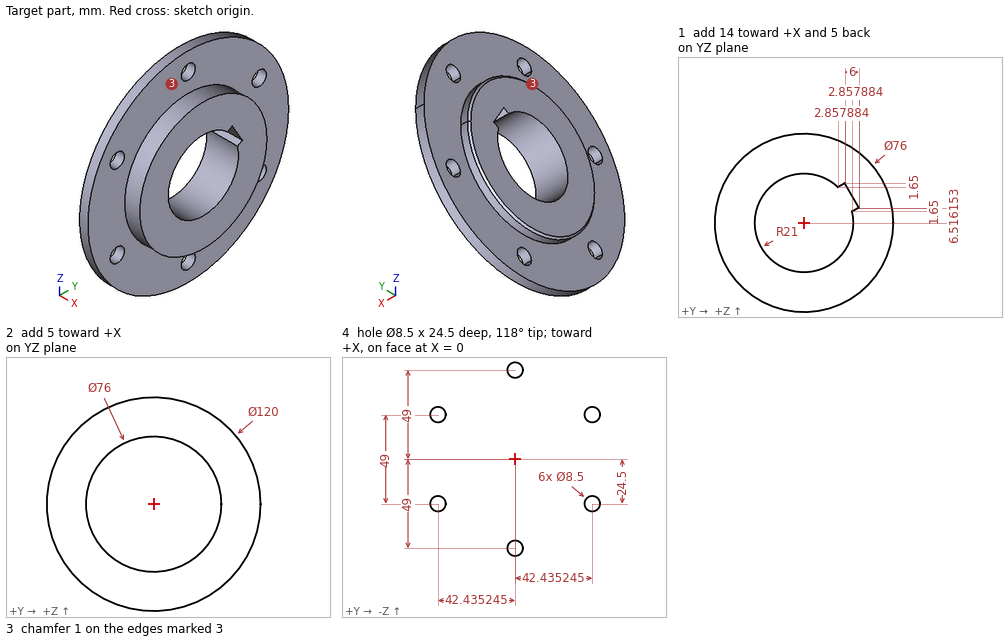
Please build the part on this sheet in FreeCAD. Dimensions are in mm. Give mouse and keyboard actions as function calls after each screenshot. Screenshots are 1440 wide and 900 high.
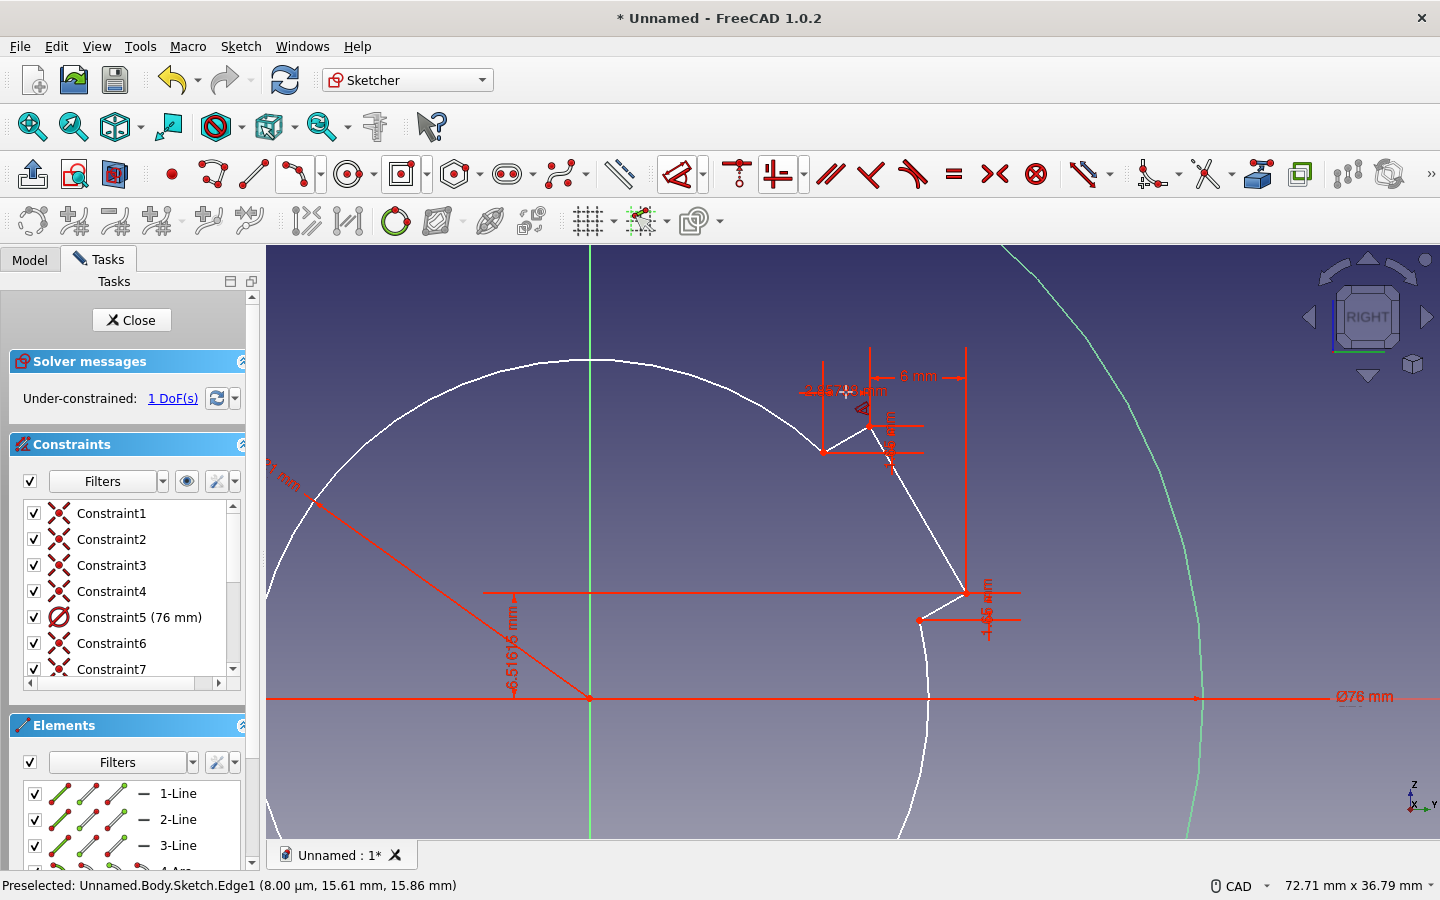
click(952, 601)
click(927, 559)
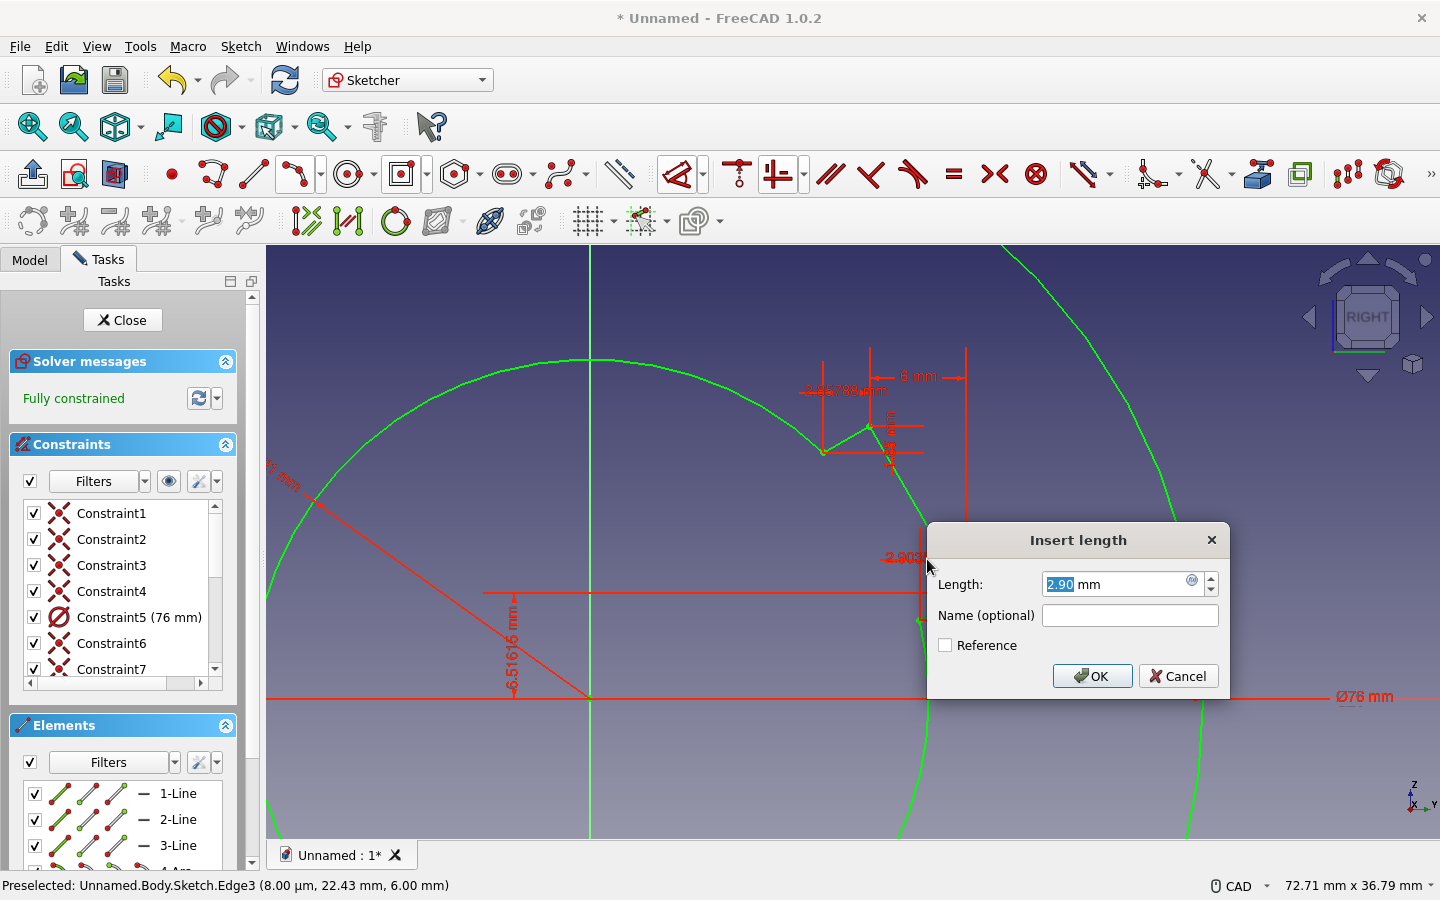
text(2.857884)
key(Return)
key(Escape)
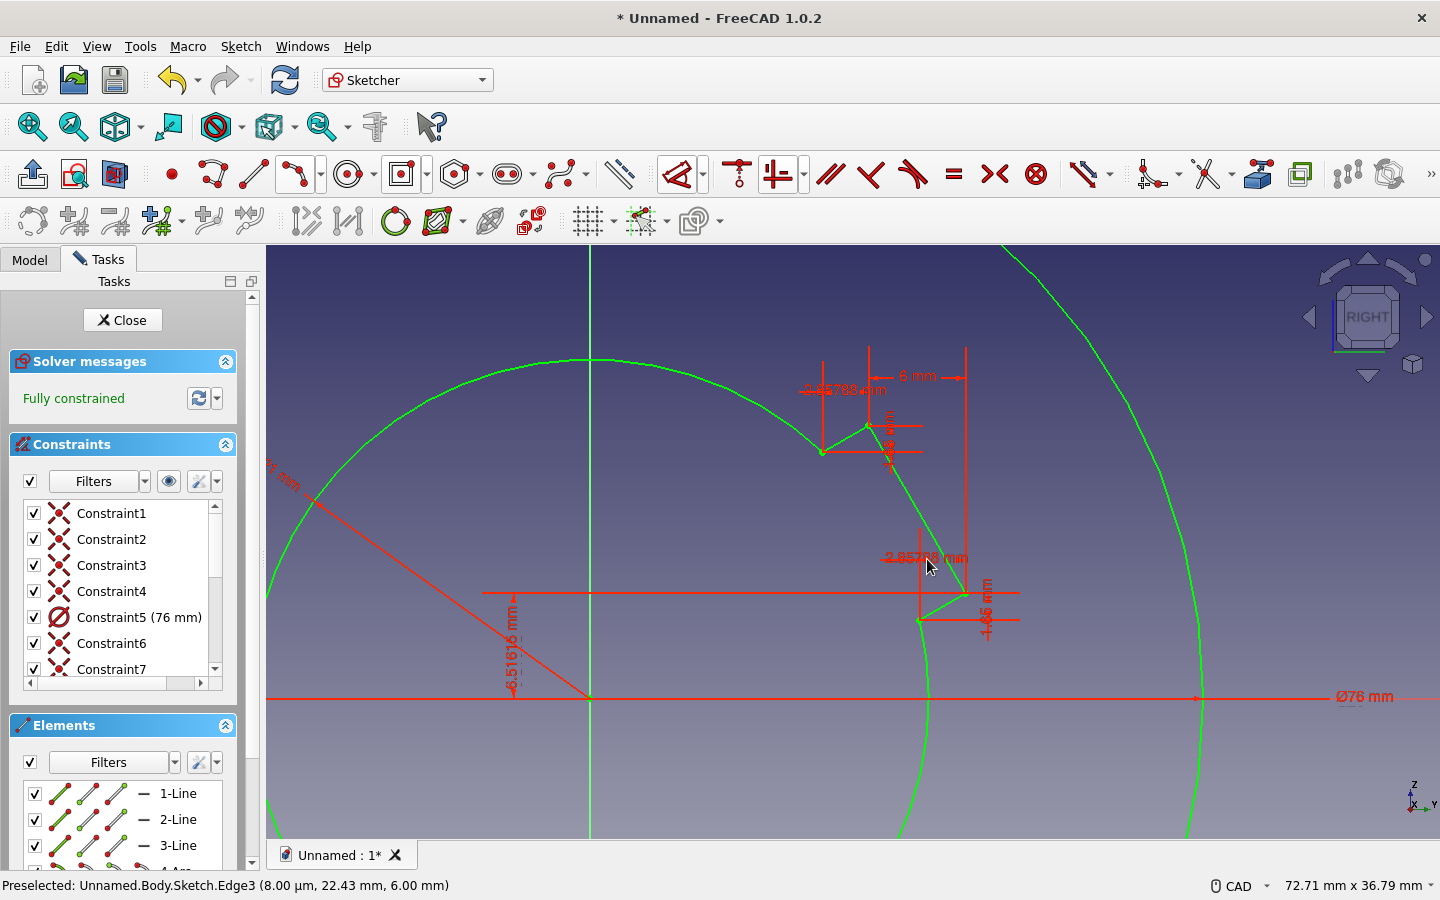
click(123, 320)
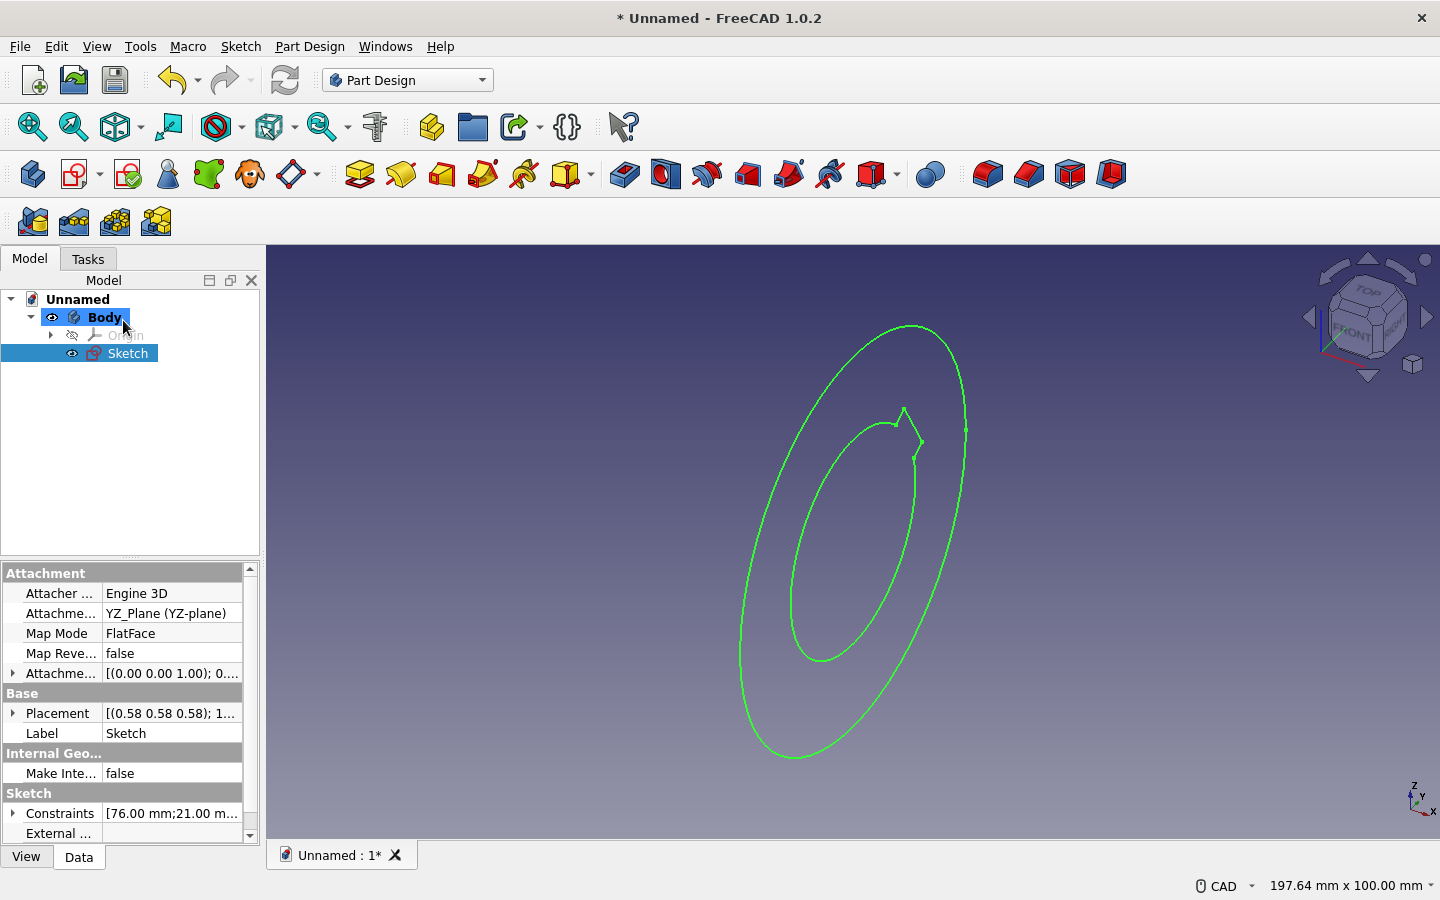
click(360, 174)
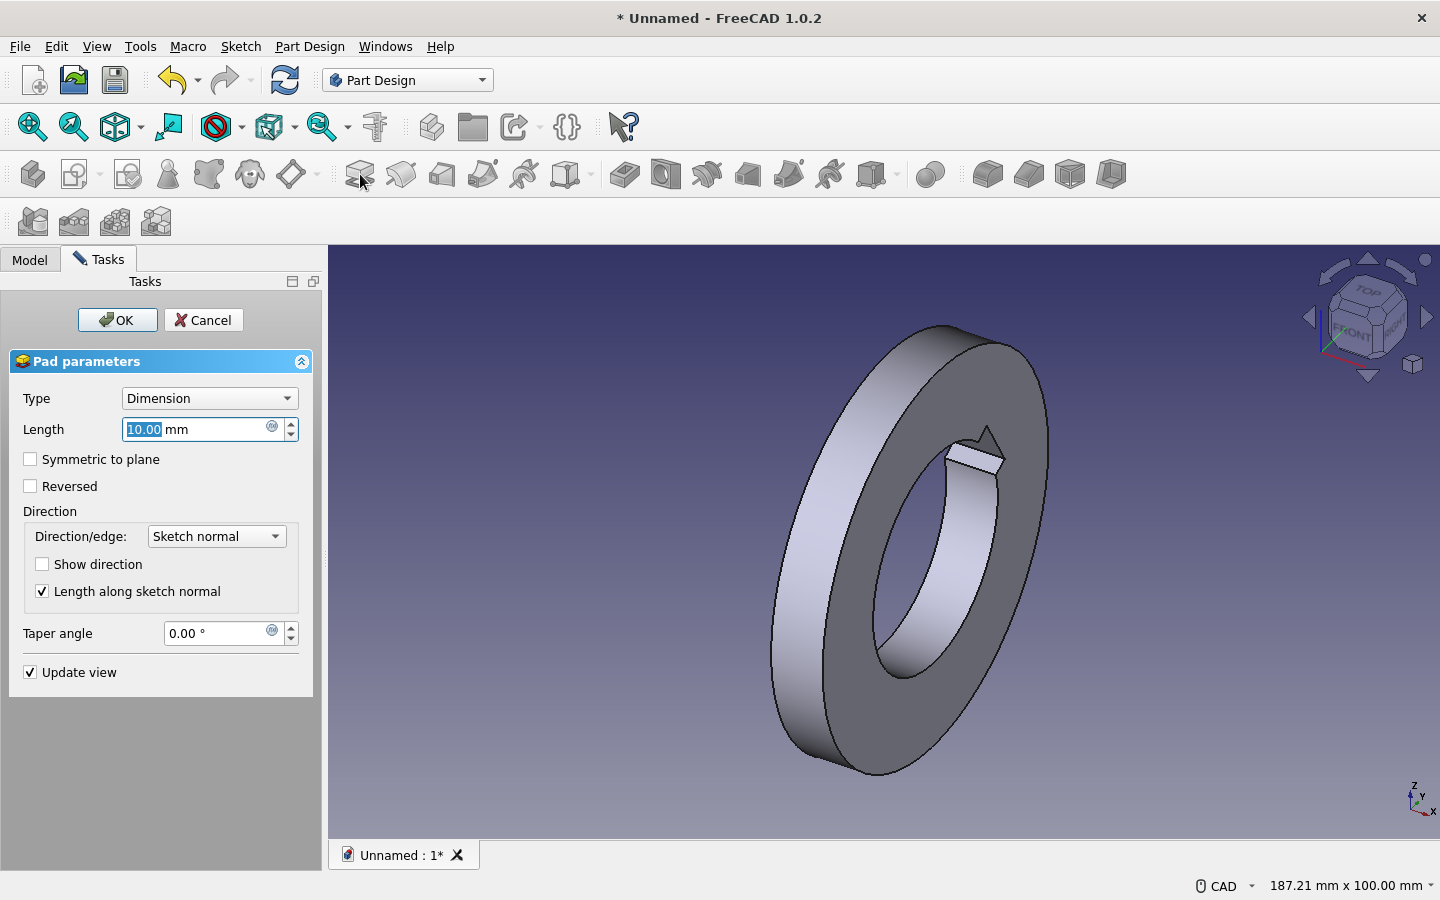
click(210, 398)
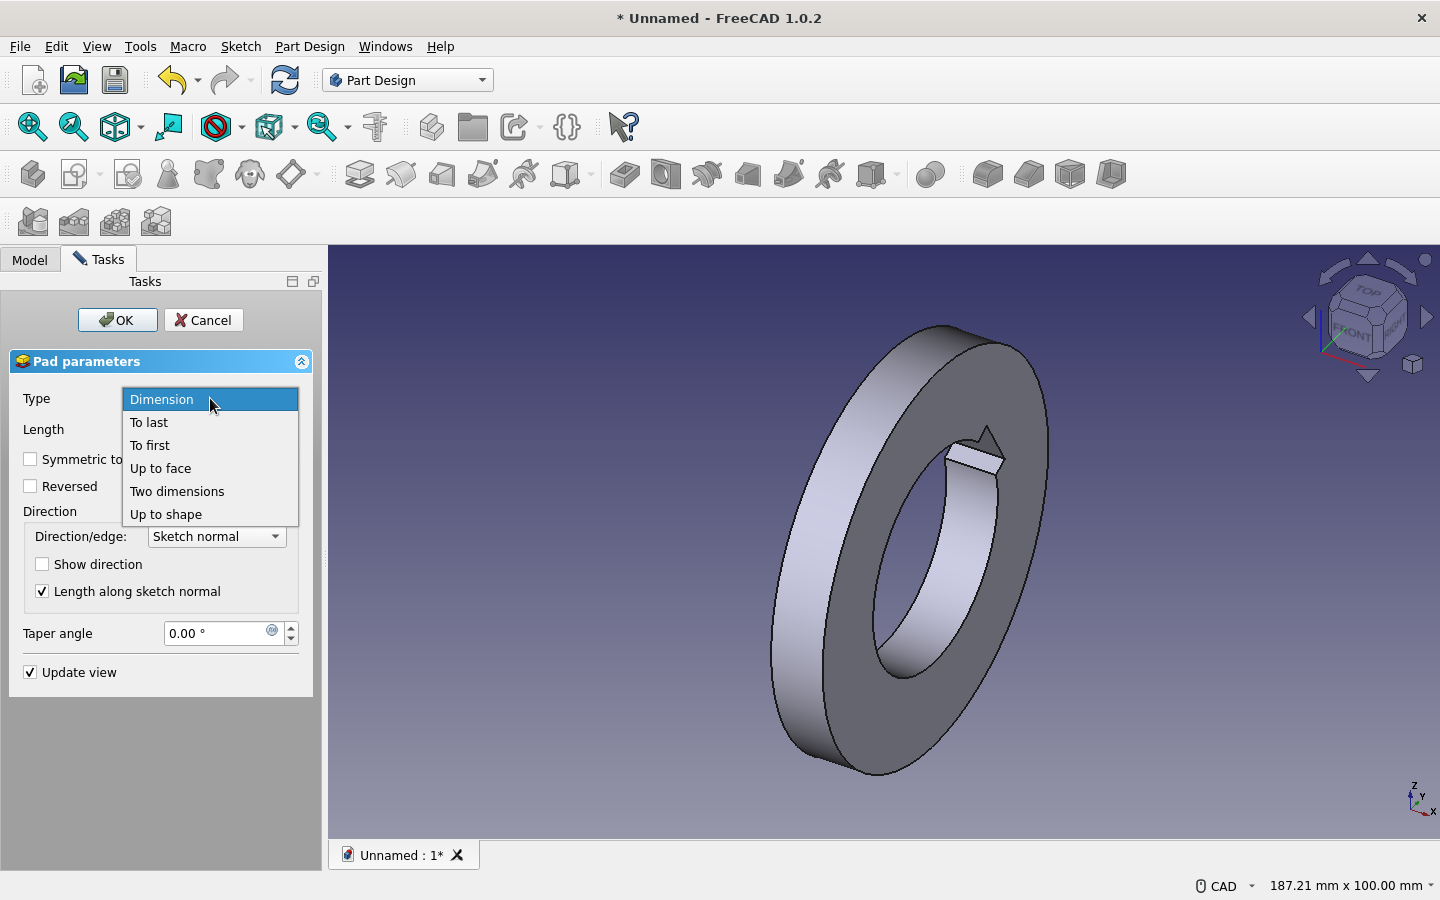
click(208, 492)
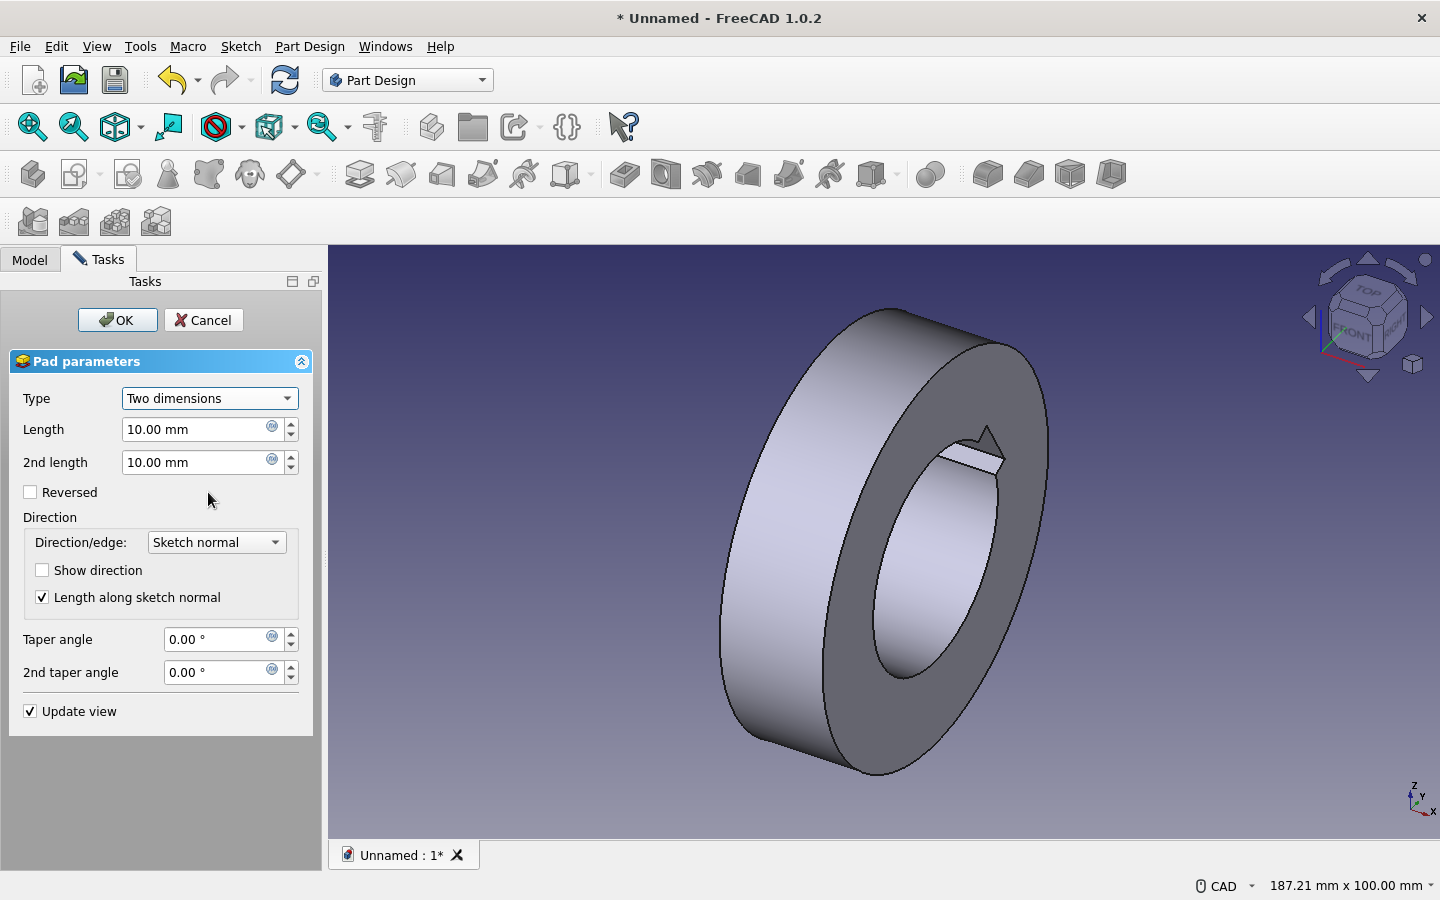
triple_click(204, 430)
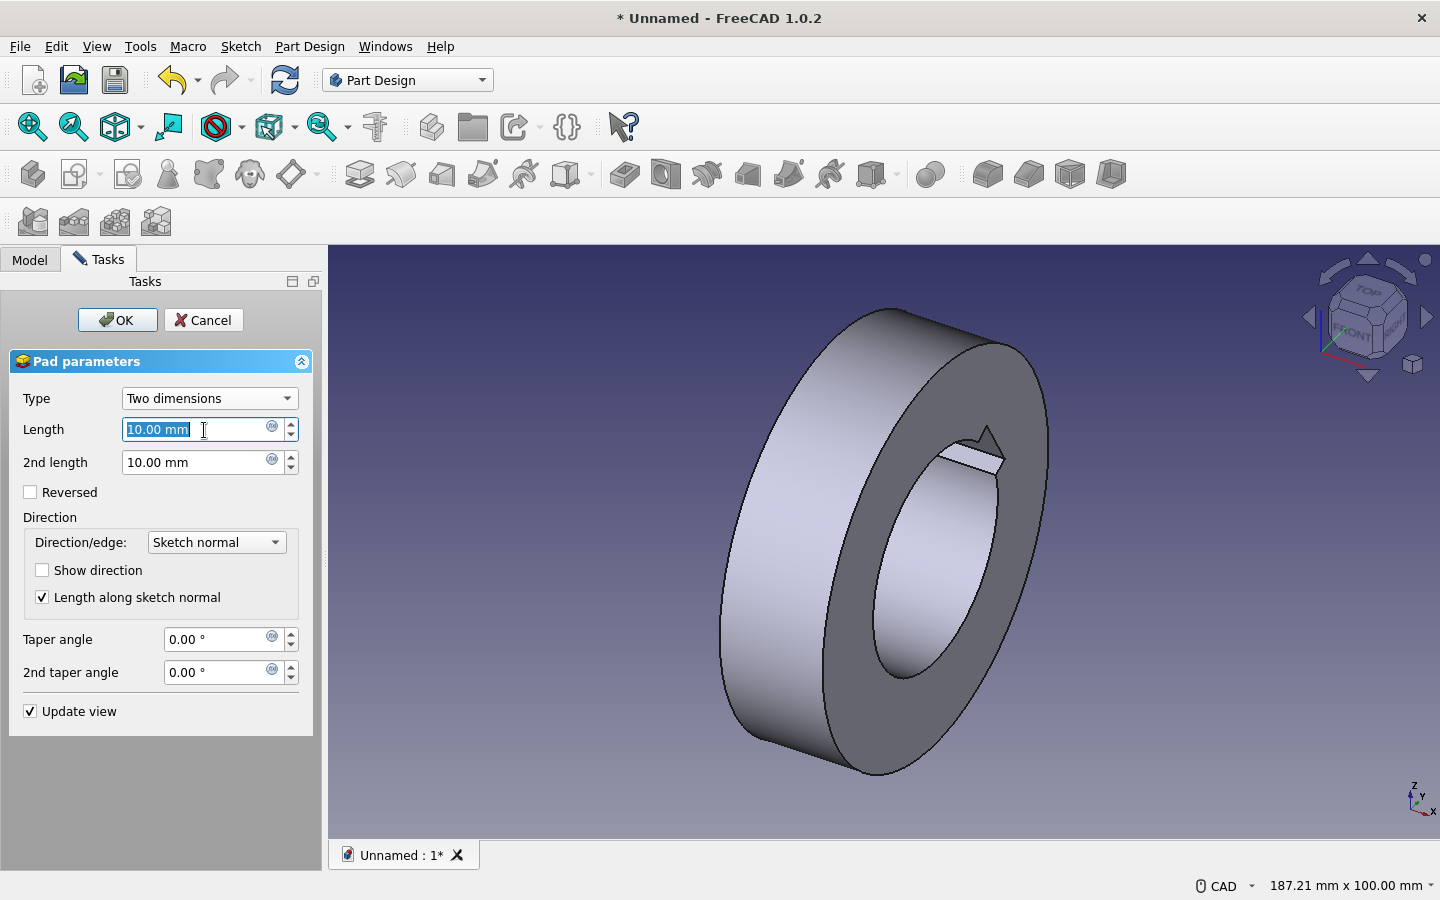
text(14)
key(Tab)